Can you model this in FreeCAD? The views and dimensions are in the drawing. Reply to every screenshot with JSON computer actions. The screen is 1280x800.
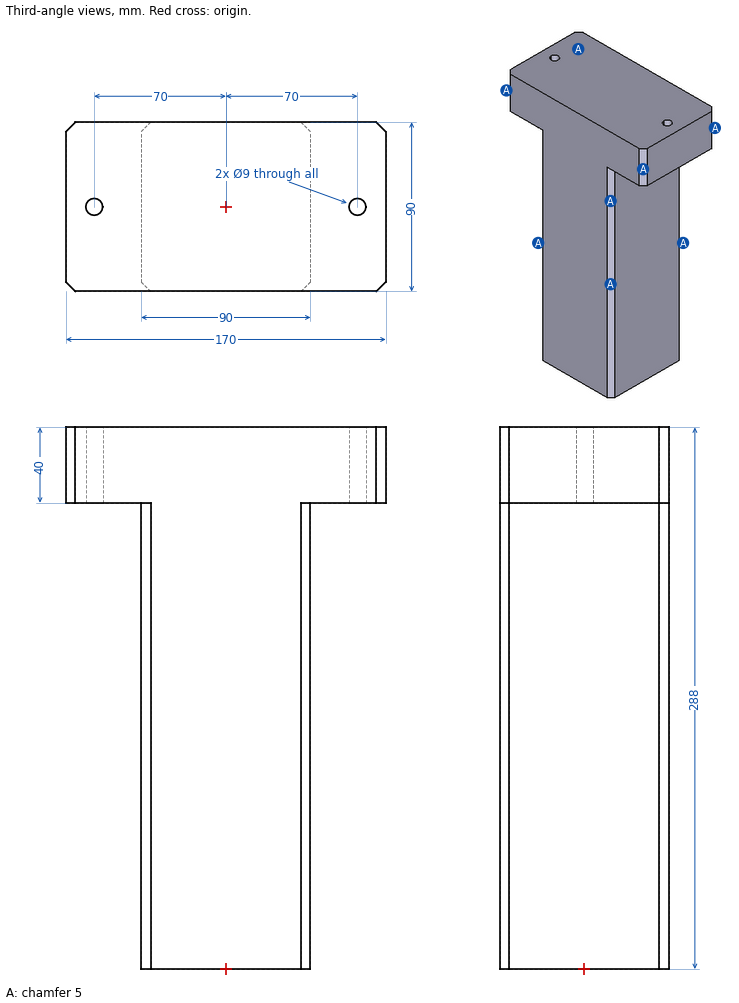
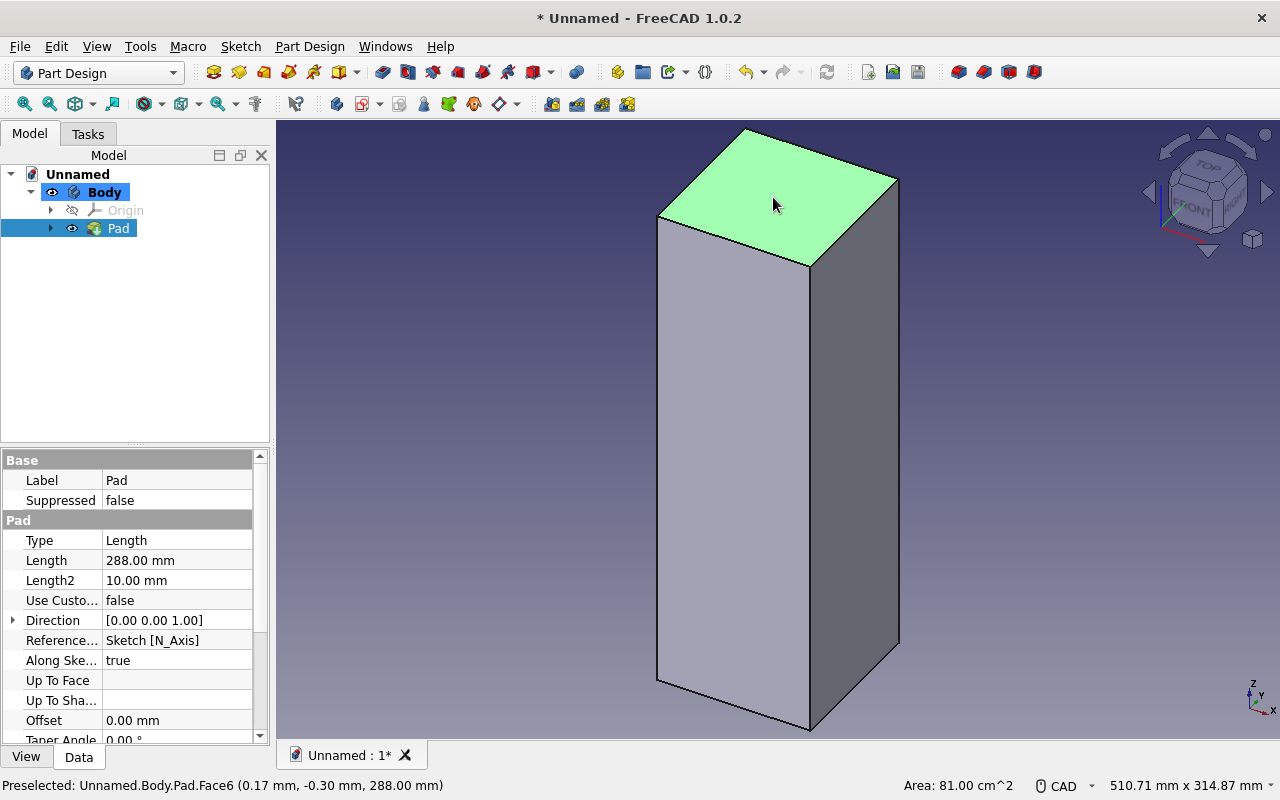
{"action": "left_click", "coordinate": [362, 104]}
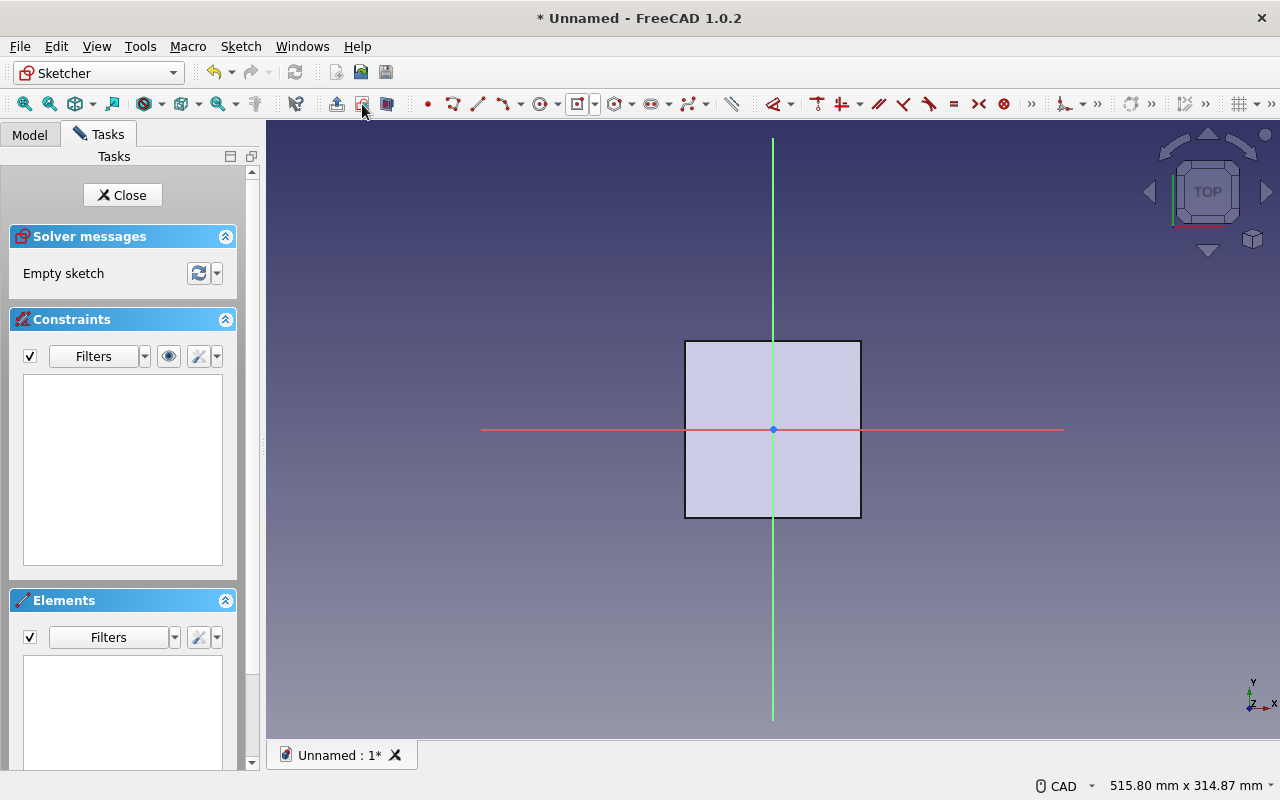
{"action": "scroll", "coordinate": [856, 430], "scroll_direction": "up", "scroll_amount": 3}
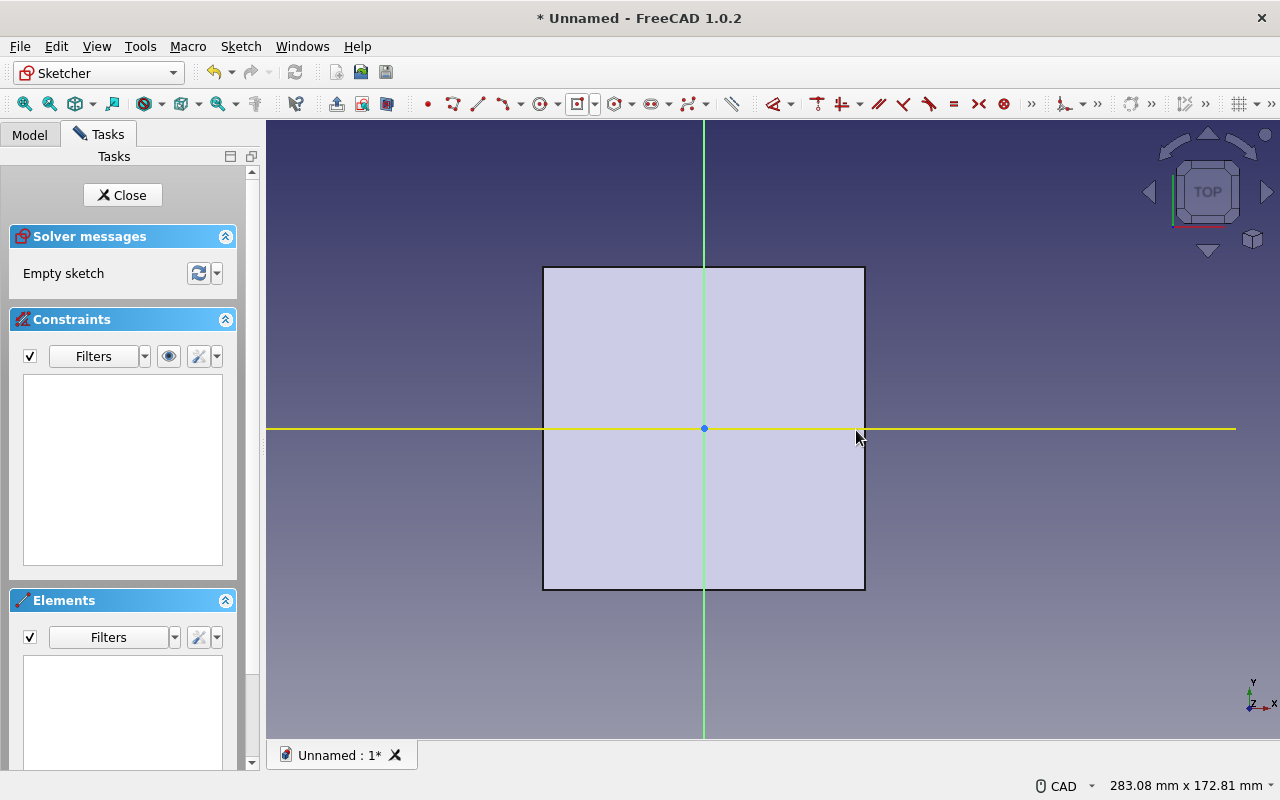
{"action": "left_click", "coordinate": [576, 104]}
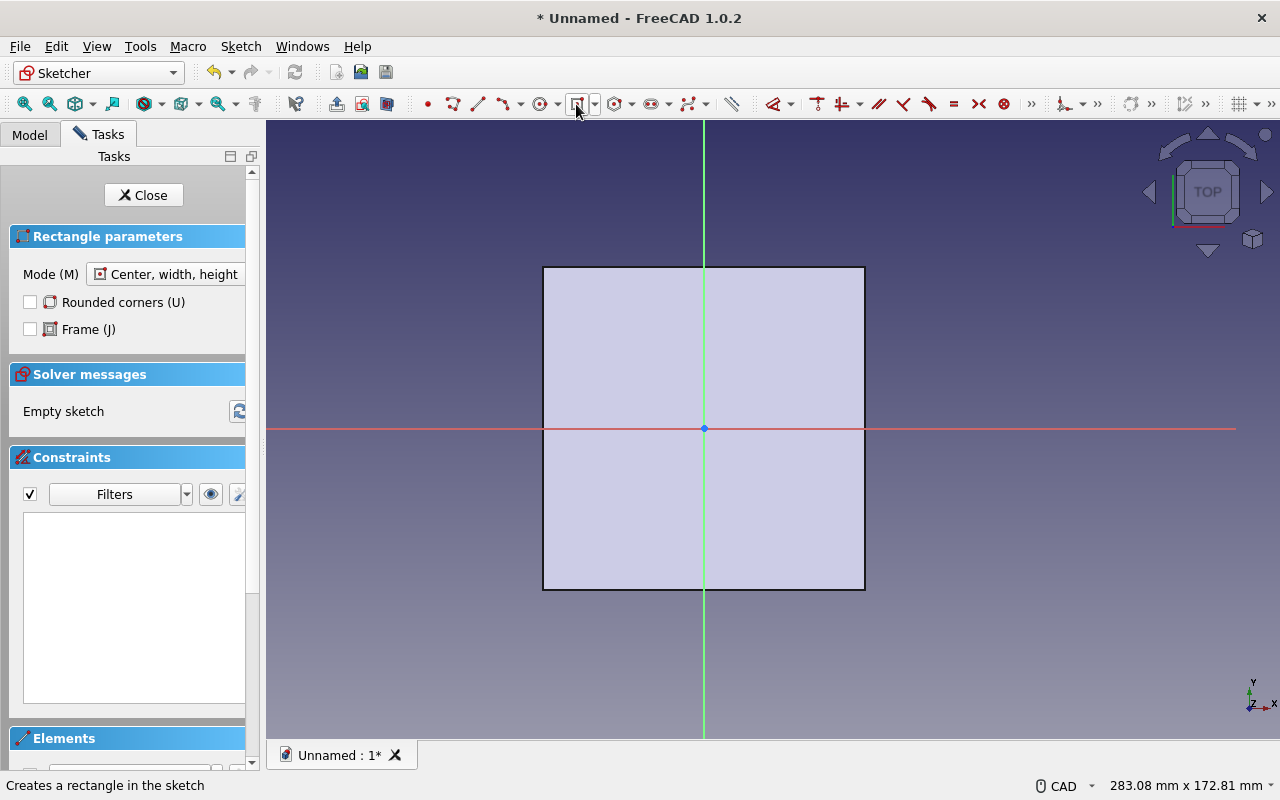
{"action": "left_click", "coordinate": [704, 429]}
{"action": "left_click", "coordinate": [1009, 267]}
{"action": "key", "text": "Escape"}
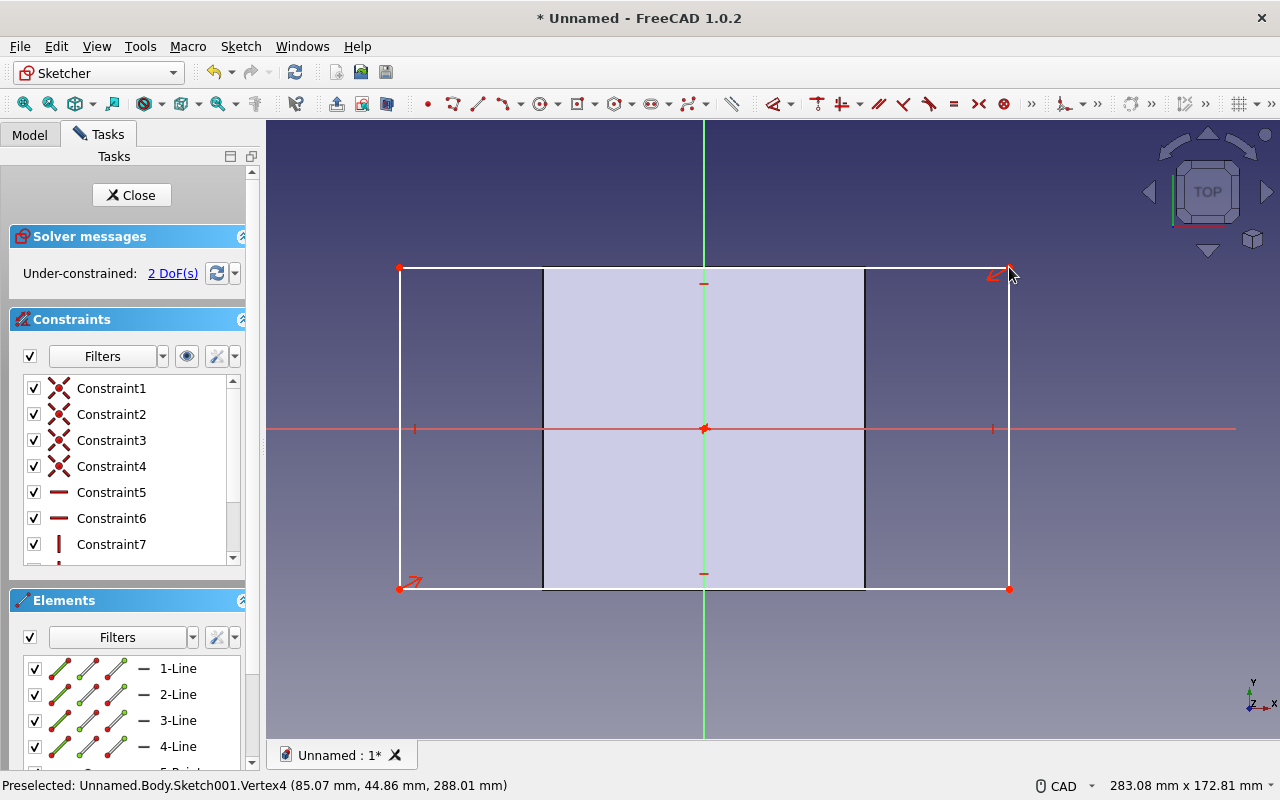
{"action": "left_click", "coordinate": [1009, 493]}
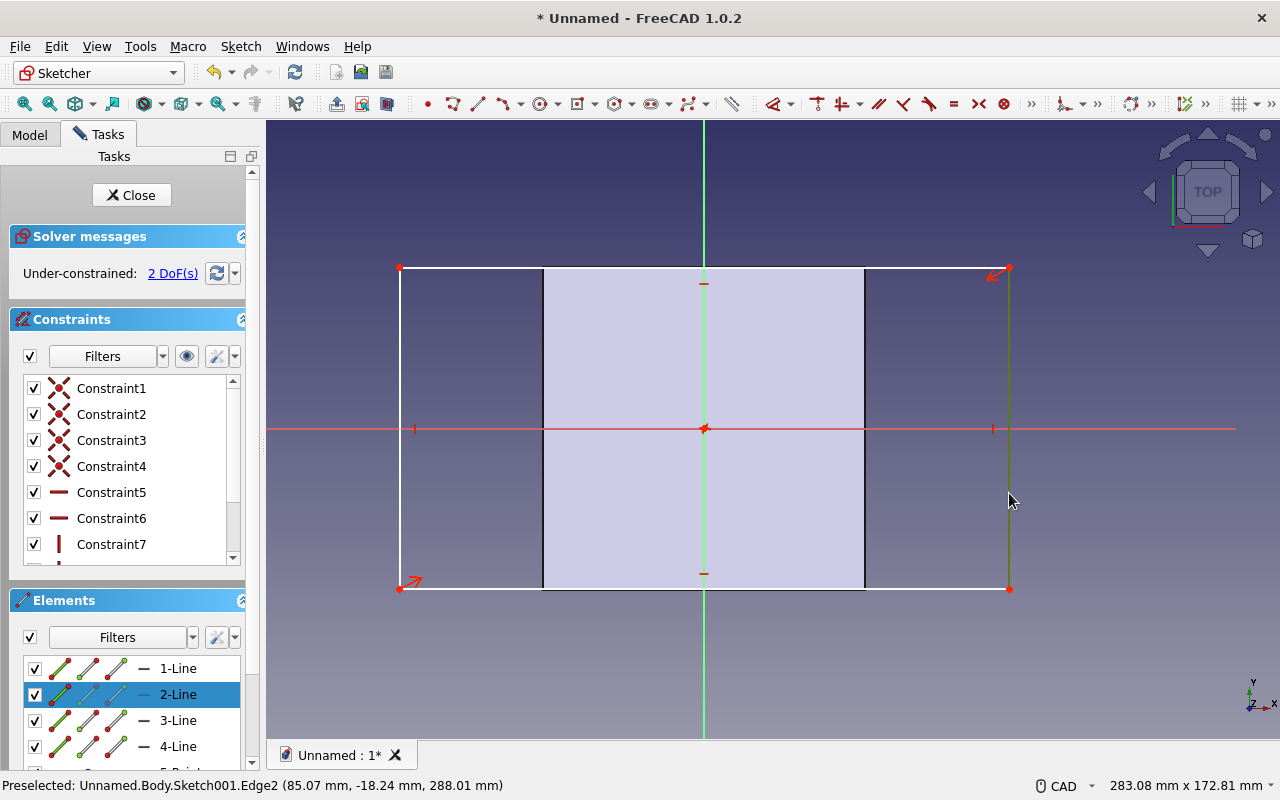
{"action": "left_click", "coordinate": [790, 104]}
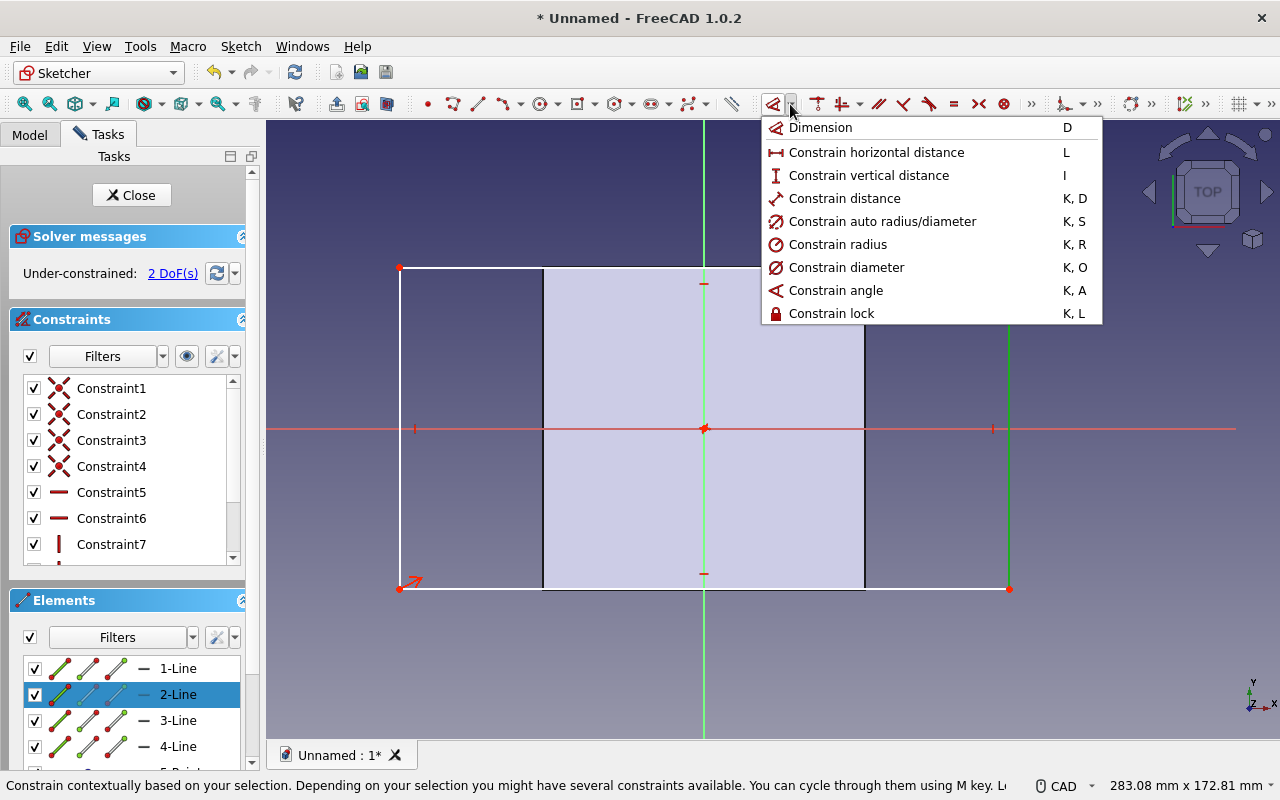
{"action": "left_click", "coordinate": [932, 176]}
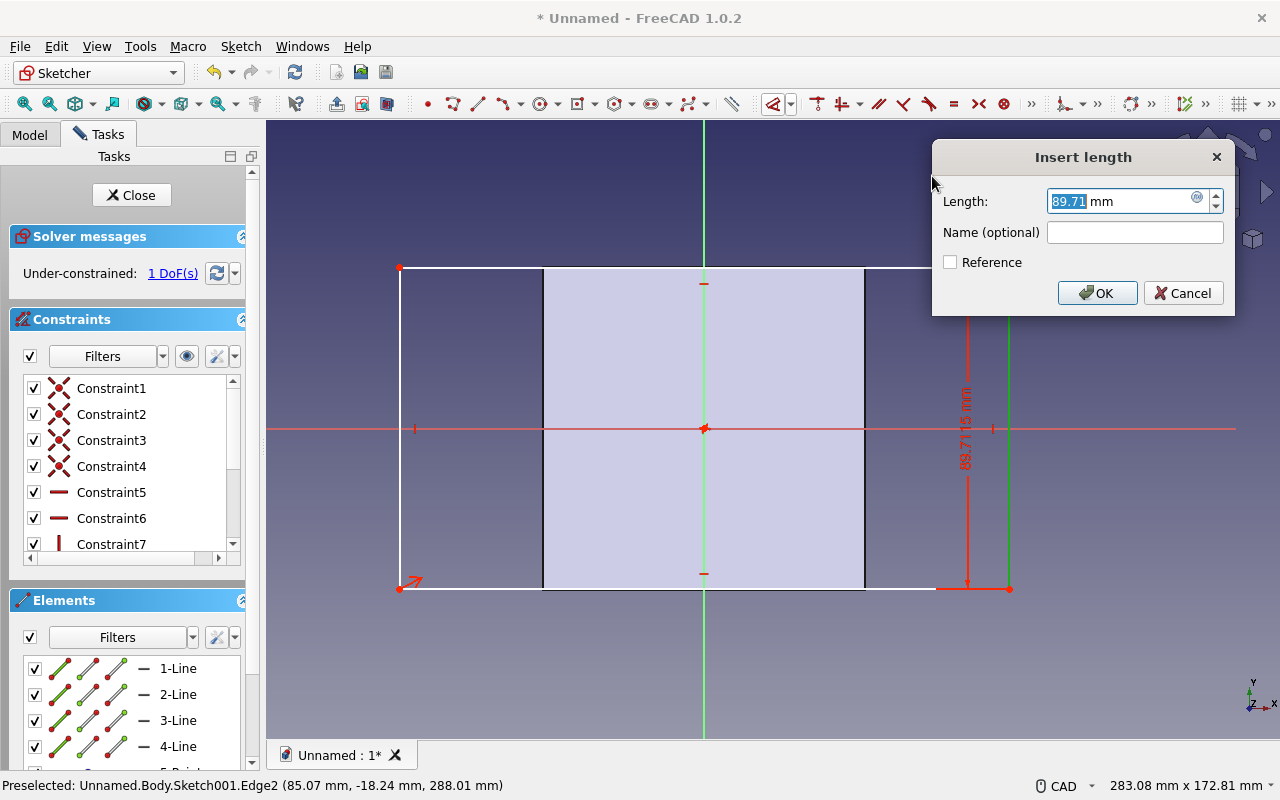
{"action": "type", "text": "90"}
{"action": "key", "text": "Return"}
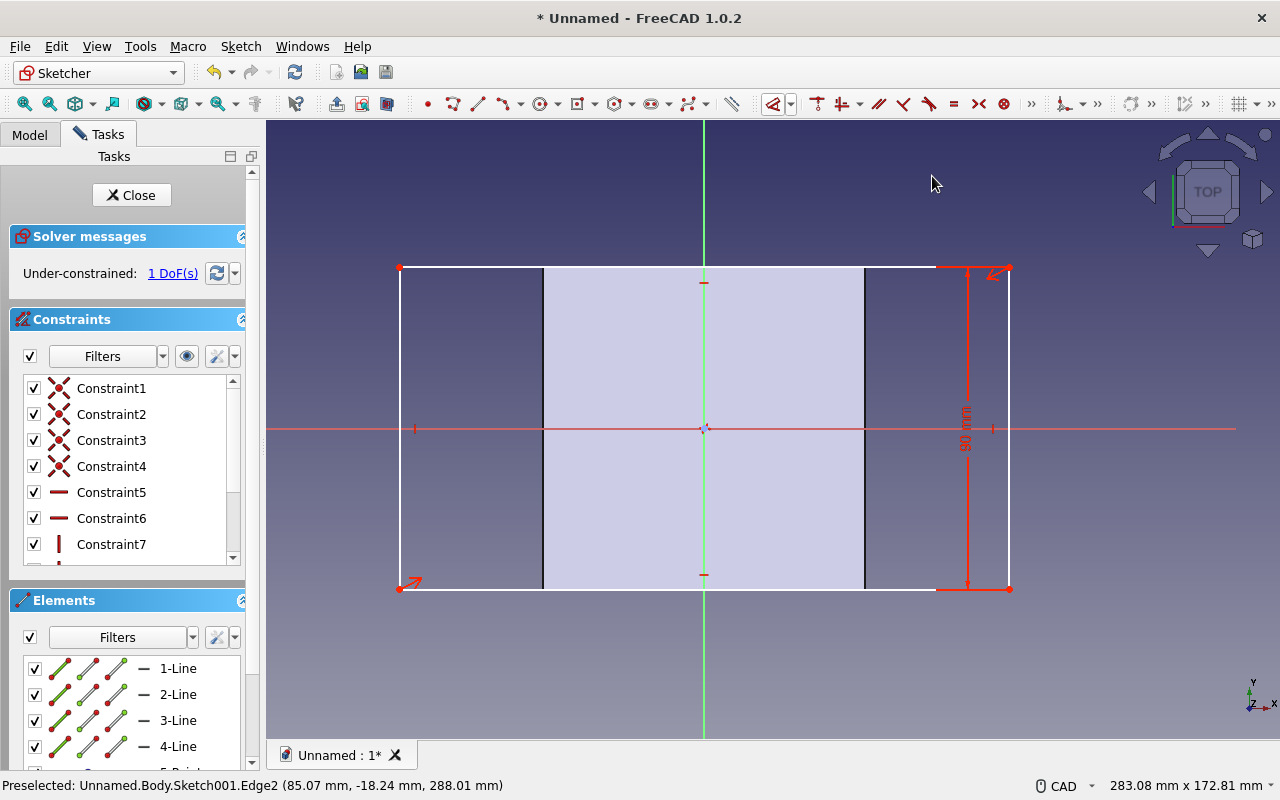
{"action": "left_click", "coordinate": [582, 590]}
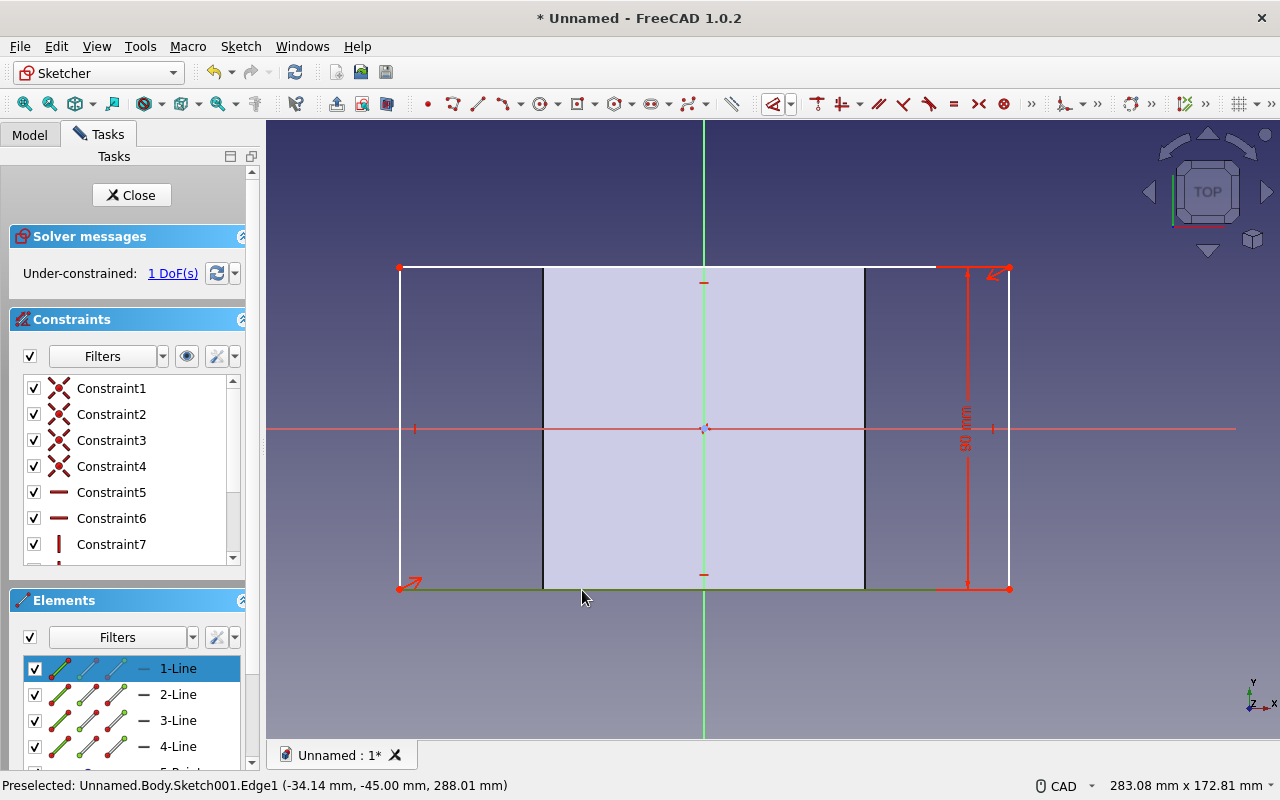
{"action": "key", "text": "l"}